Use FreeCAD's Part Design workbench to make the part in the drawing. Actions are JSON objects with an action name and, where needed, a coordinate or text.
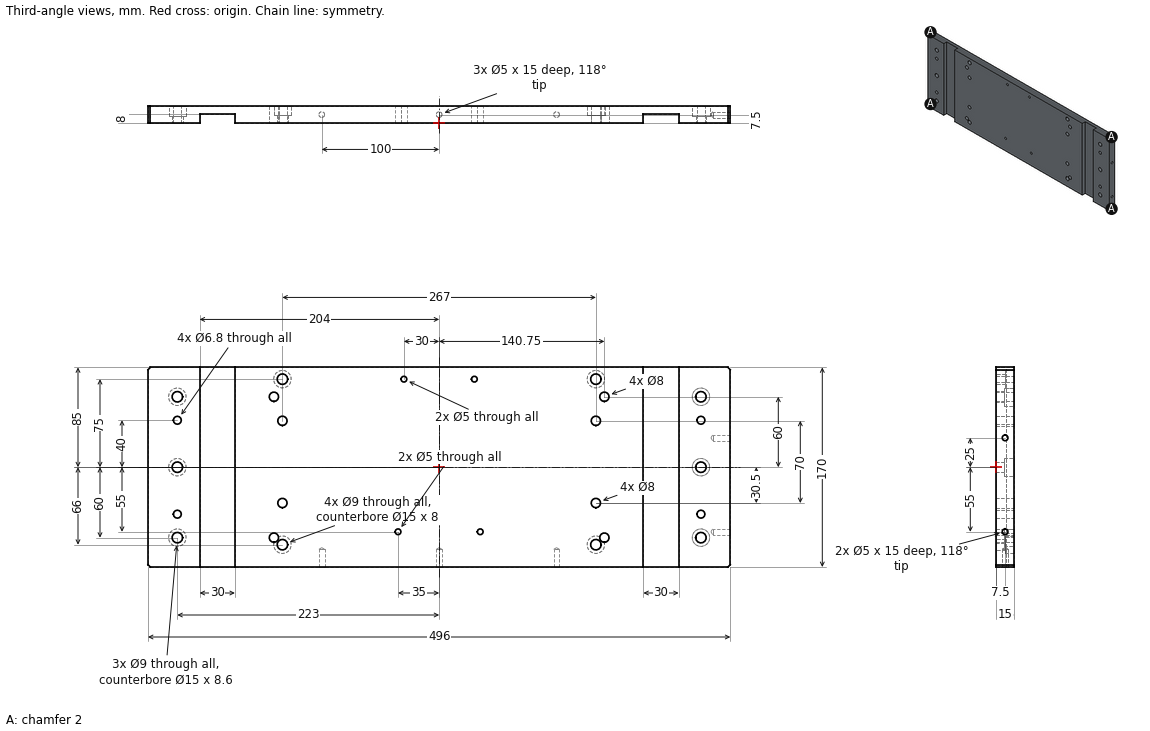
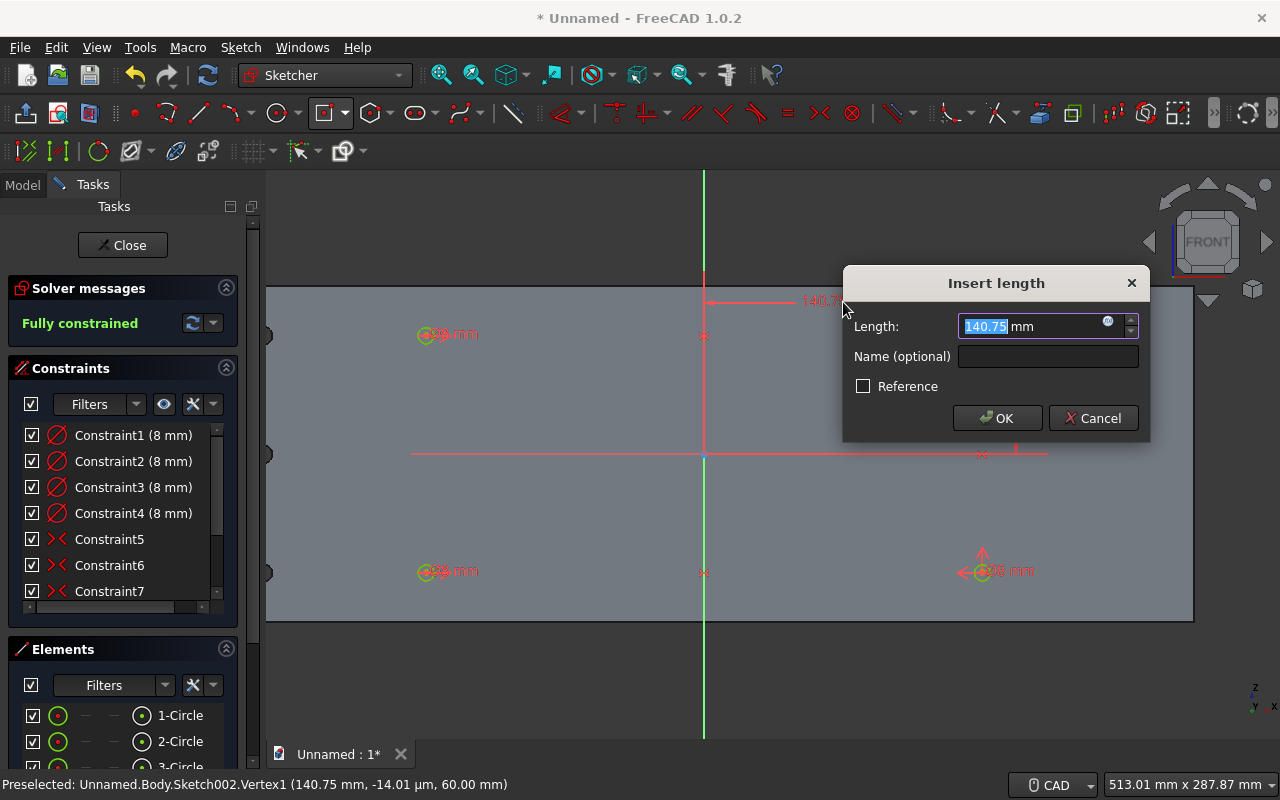
{"action": "type", "text": "140.75"}
{"action": "key", "text": "Return"}
{"action": "key", "text": "Escape"}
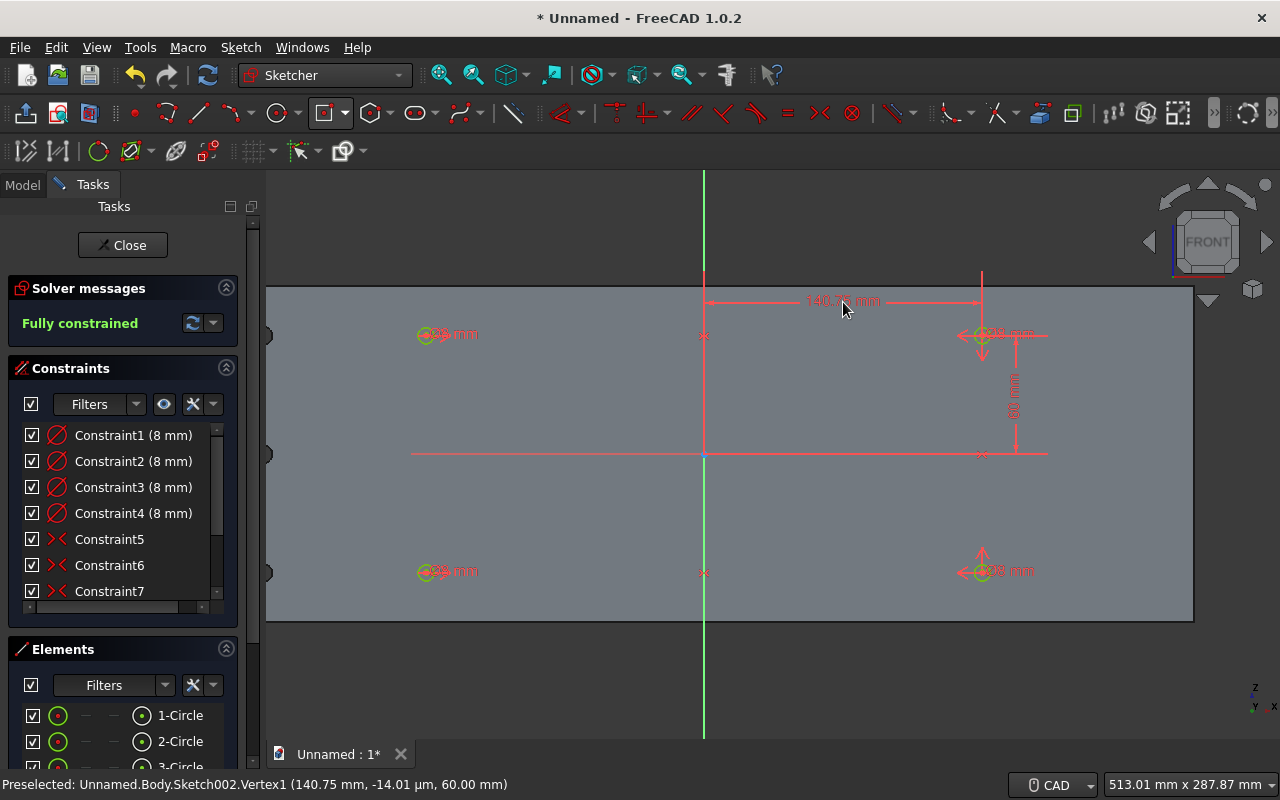
{"action": "left_click", "coordinate": [123, 245]}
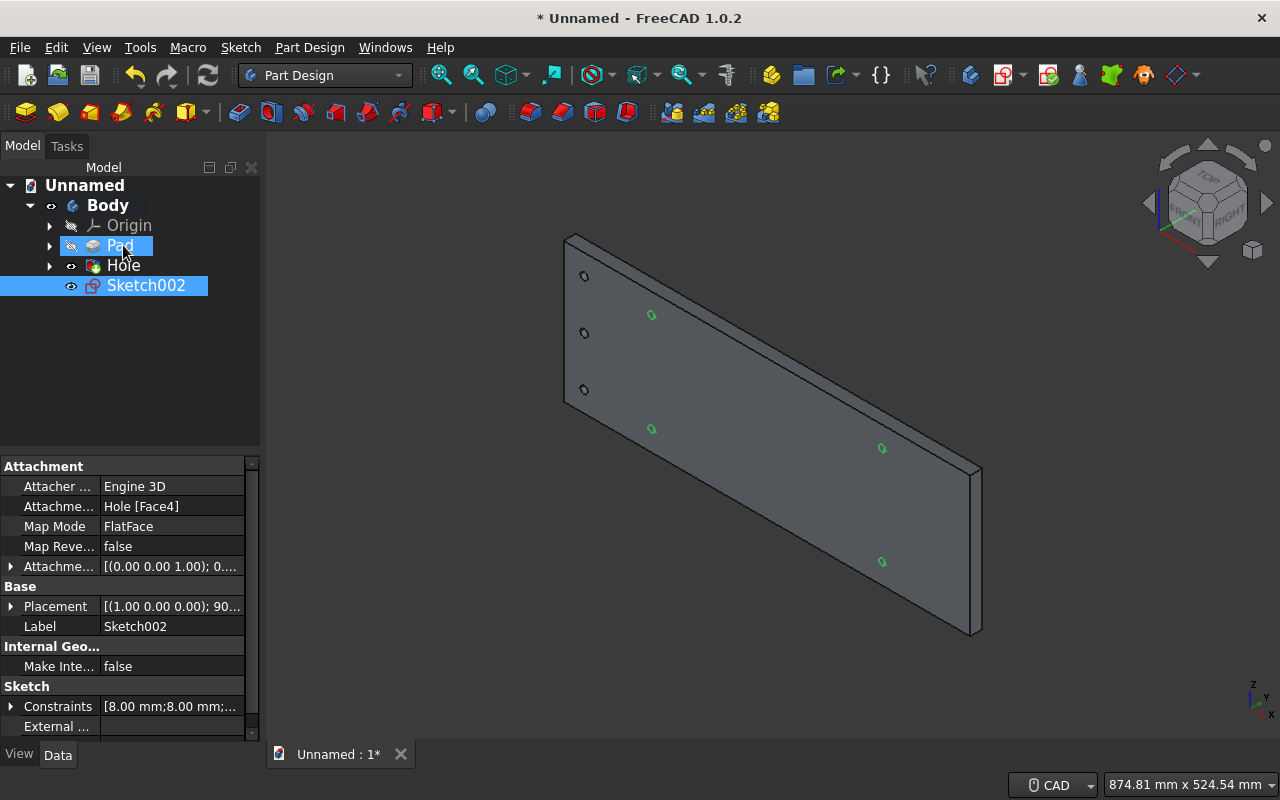
{"action": "left_click", "coordinate": [240, 112]}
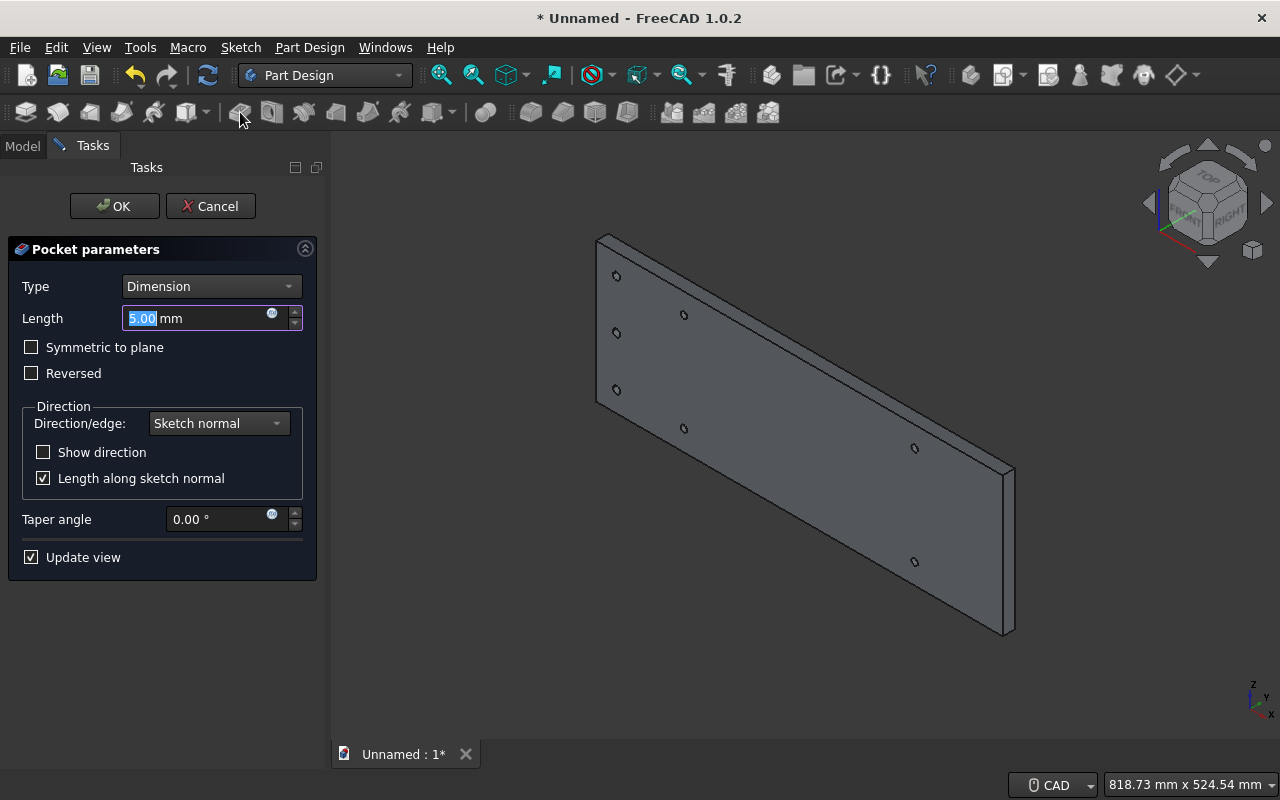
{"action": "left_click", "coordinate": [212, 286]}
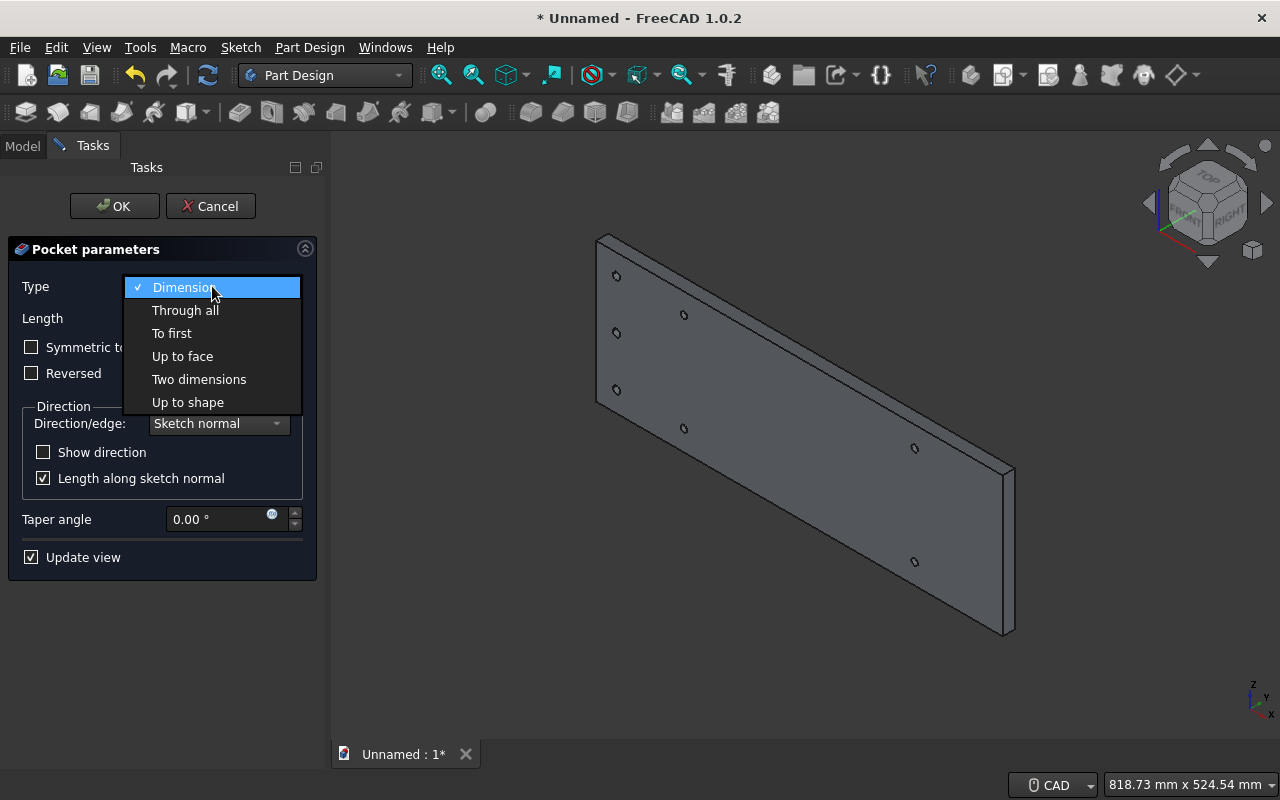
{"action": "left_click", "coordinate": [212, 310]}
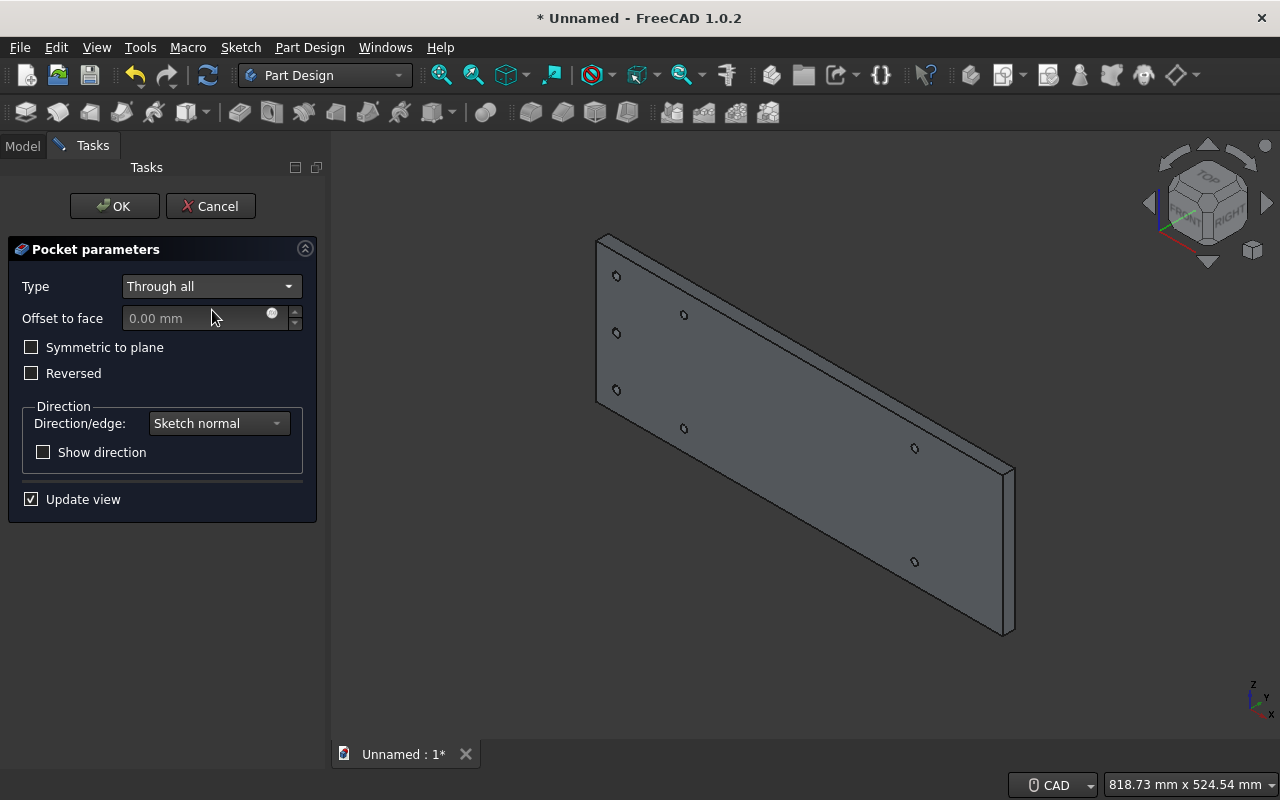
{"action": "left_click", "coordinate": [115, 206]}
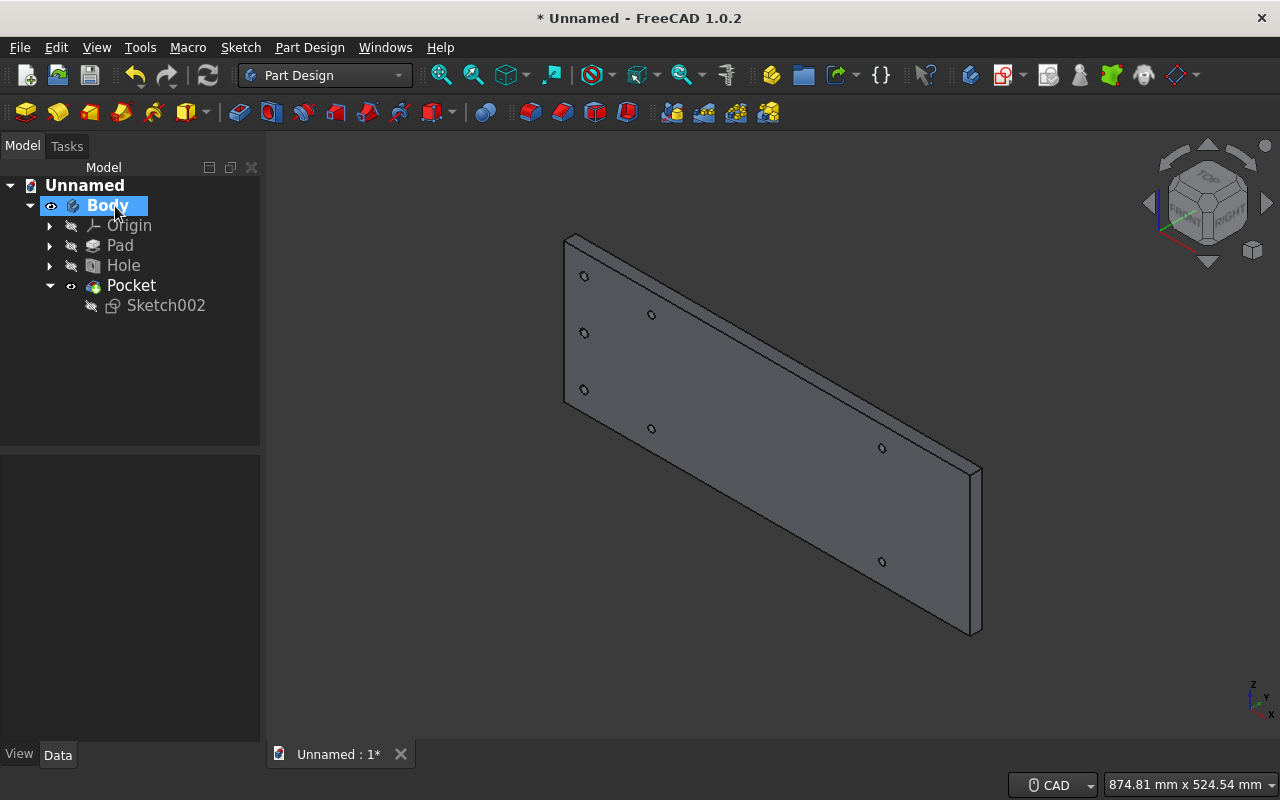
{"action": "left_click", "coordinate": [1004, 76]}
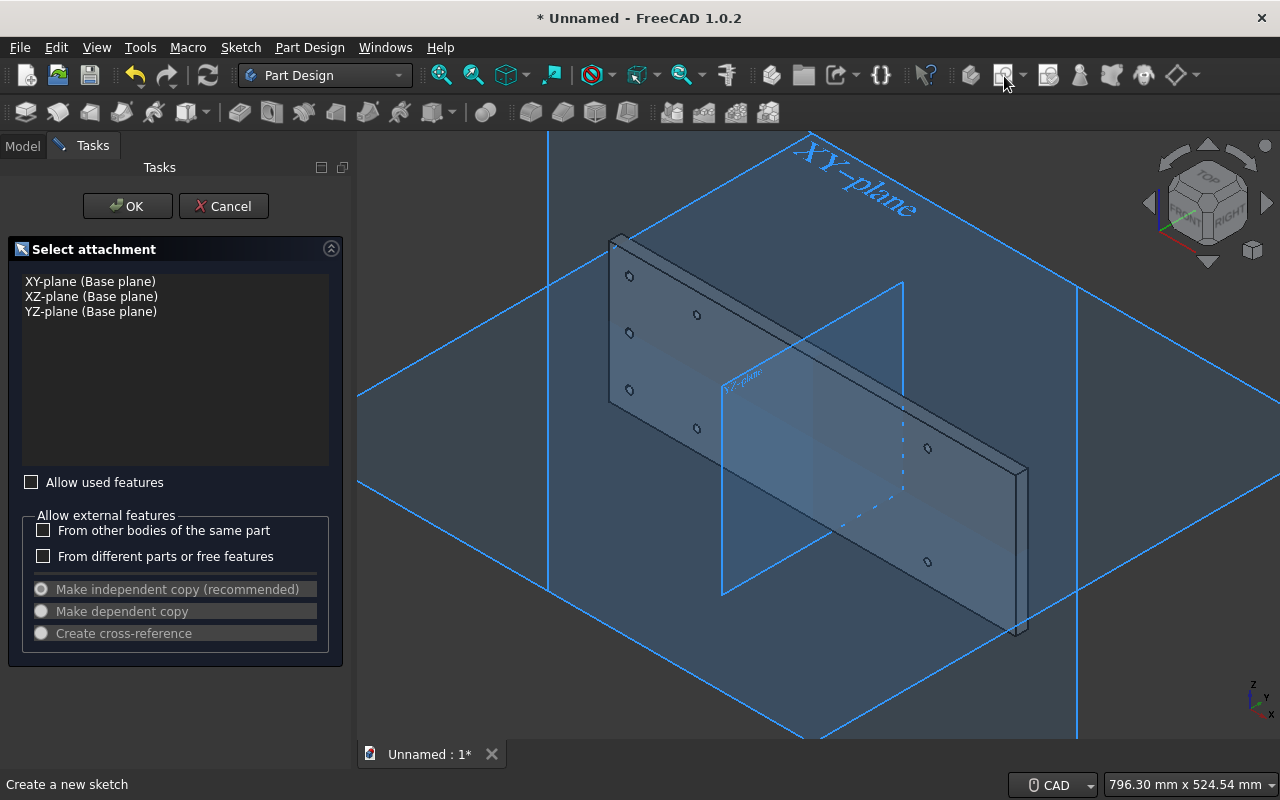
{"action": "left_click", "coordinate": [82, 296]}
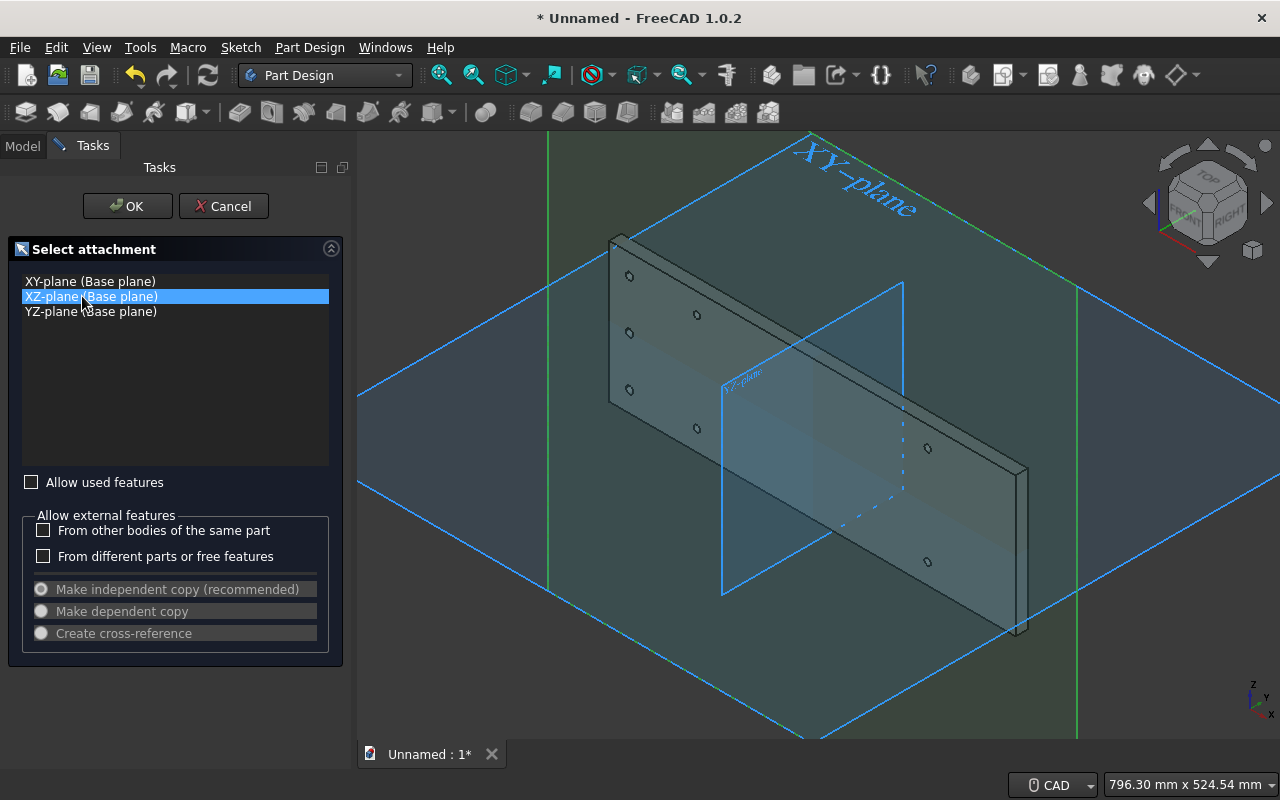
{"action": "left_click", "coordinate": [128, 206]}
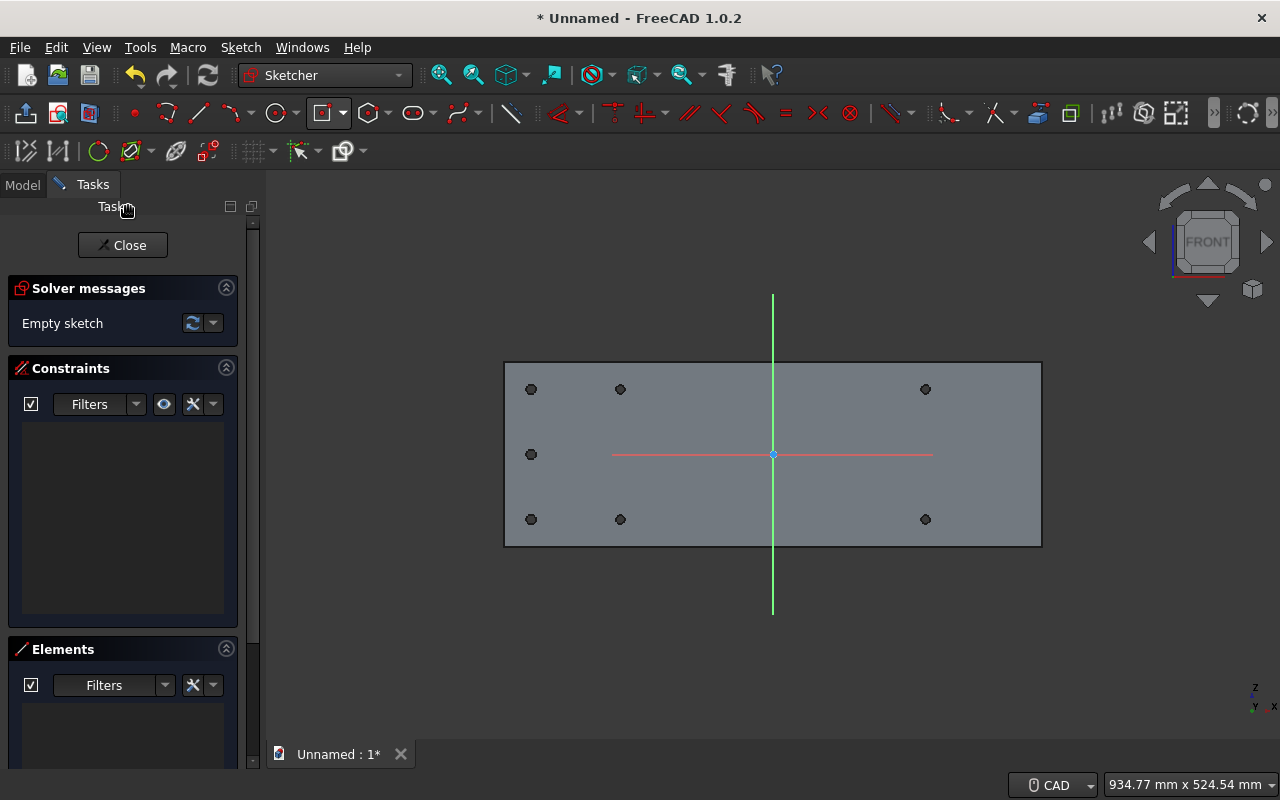
{"action": "scroll", "coordinate": [856, 444], "scroll_direction": "up", "scroll_amount": 3}